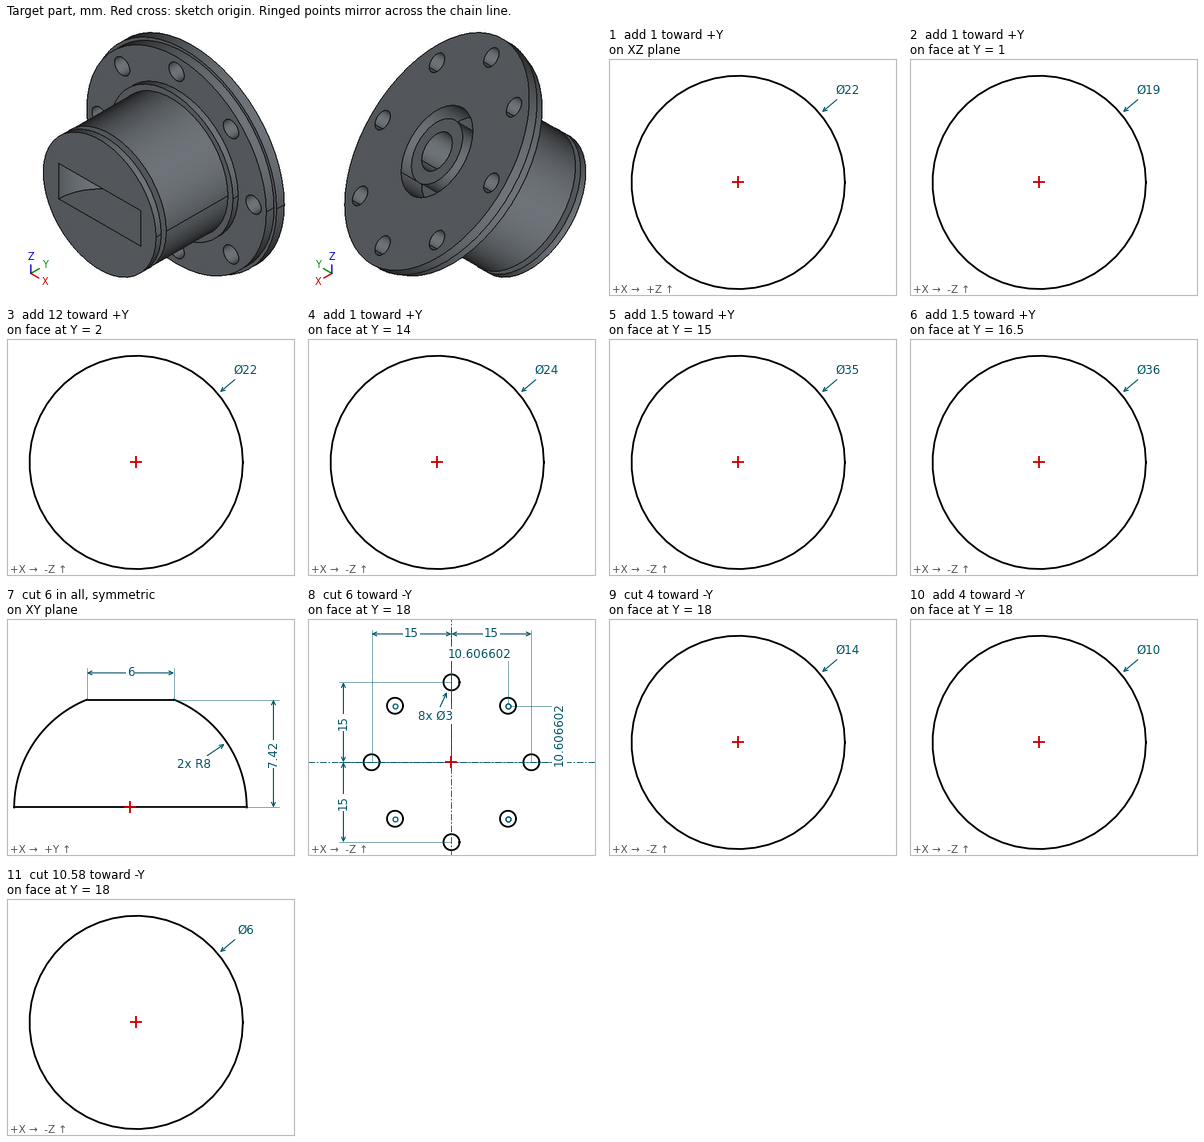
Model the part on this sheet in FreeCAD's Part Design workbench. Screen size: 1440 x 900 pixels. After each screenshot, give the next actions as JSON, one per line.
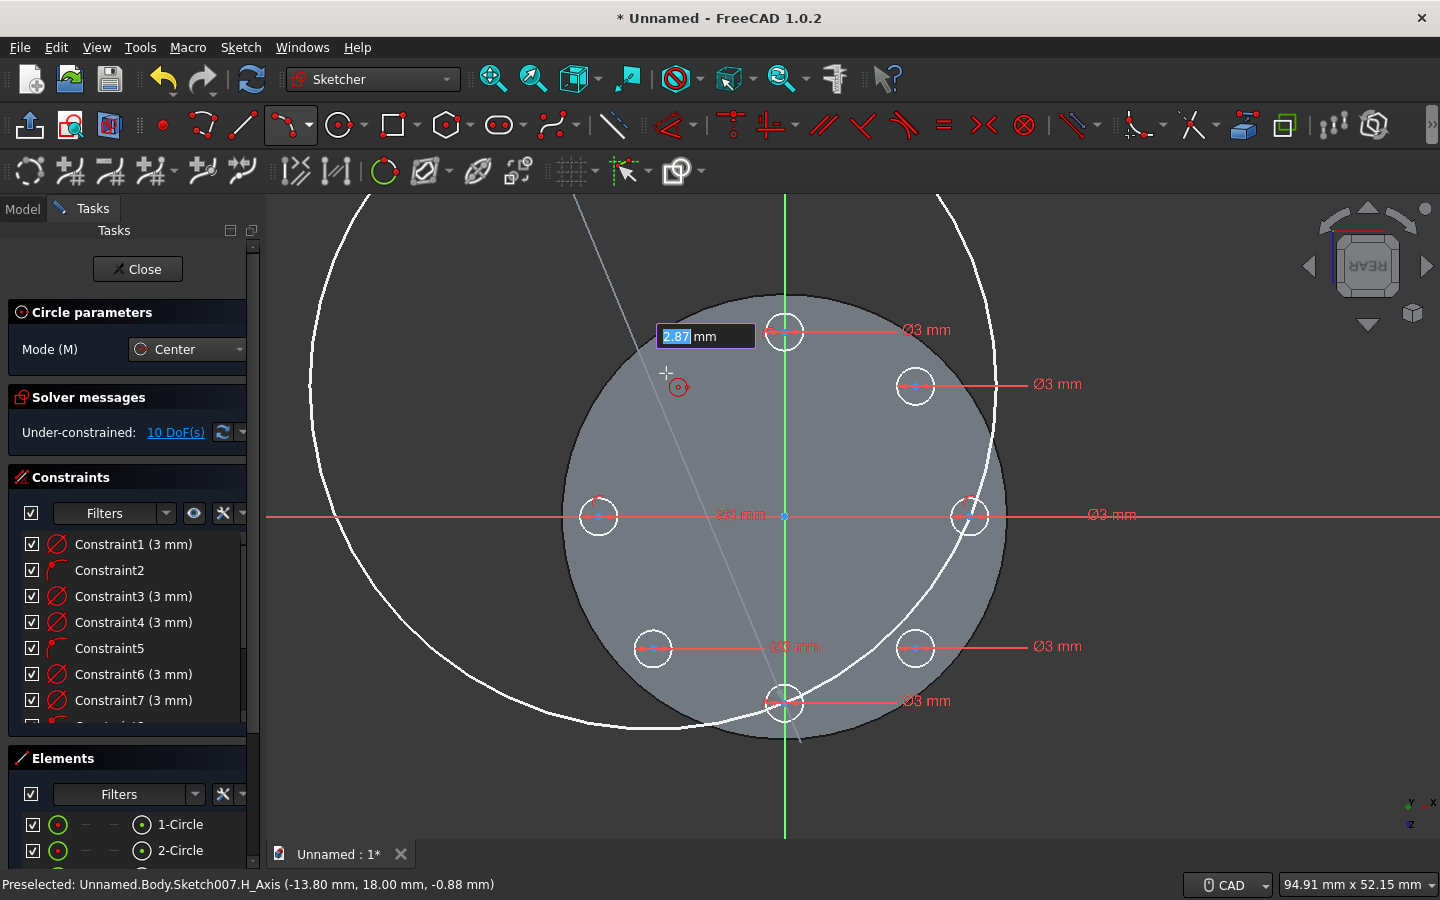
{"action": "type", "text": "3"}
{"action": "key", "text": "Return"}
{"action": "key", "text": "Escape"}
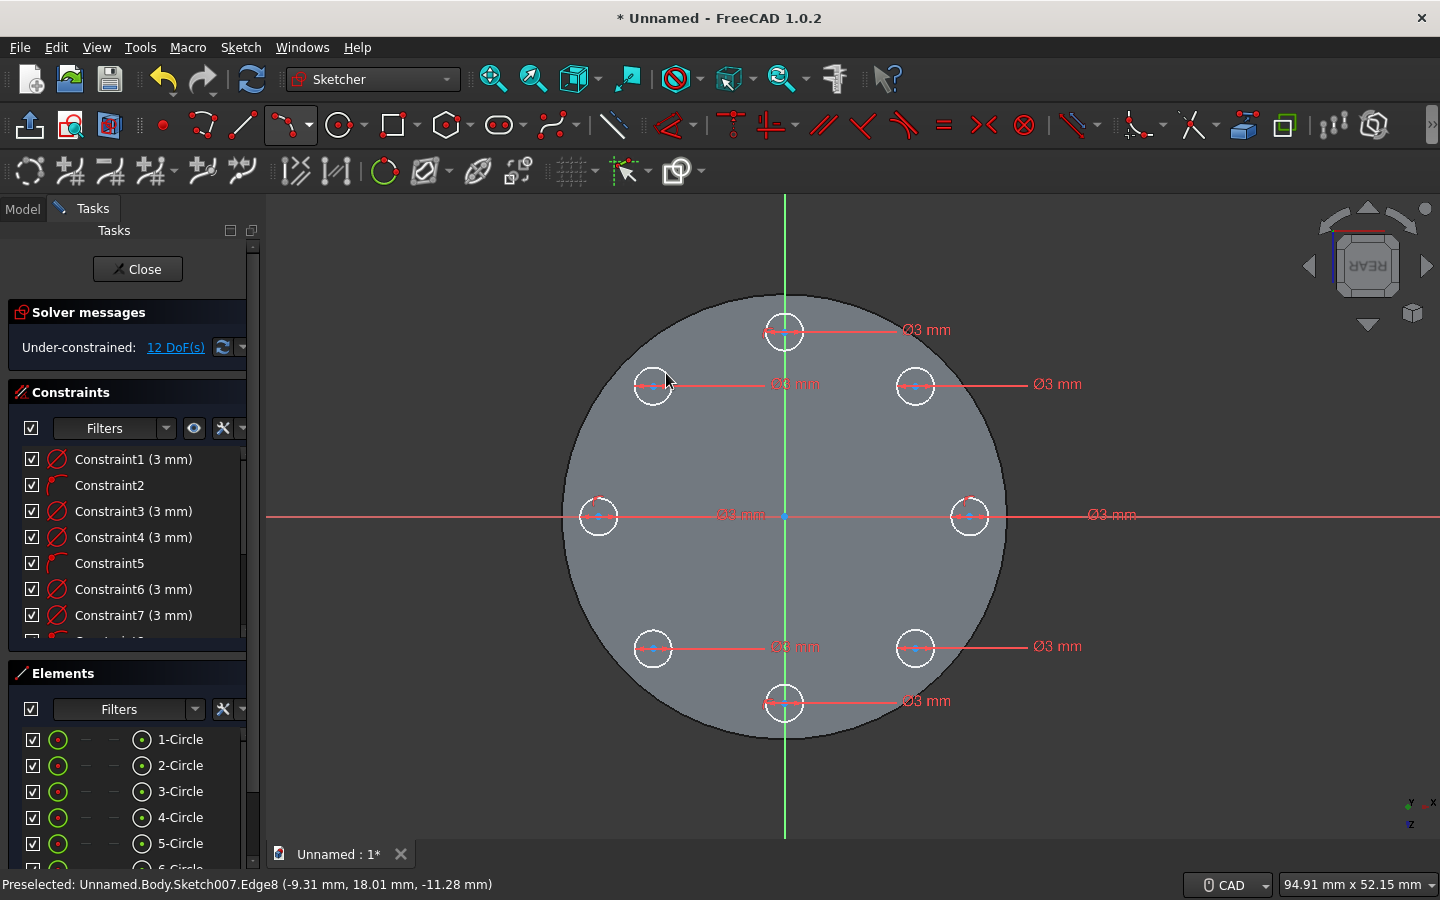
{"action": "left_click", "coordinate": [916, 386]}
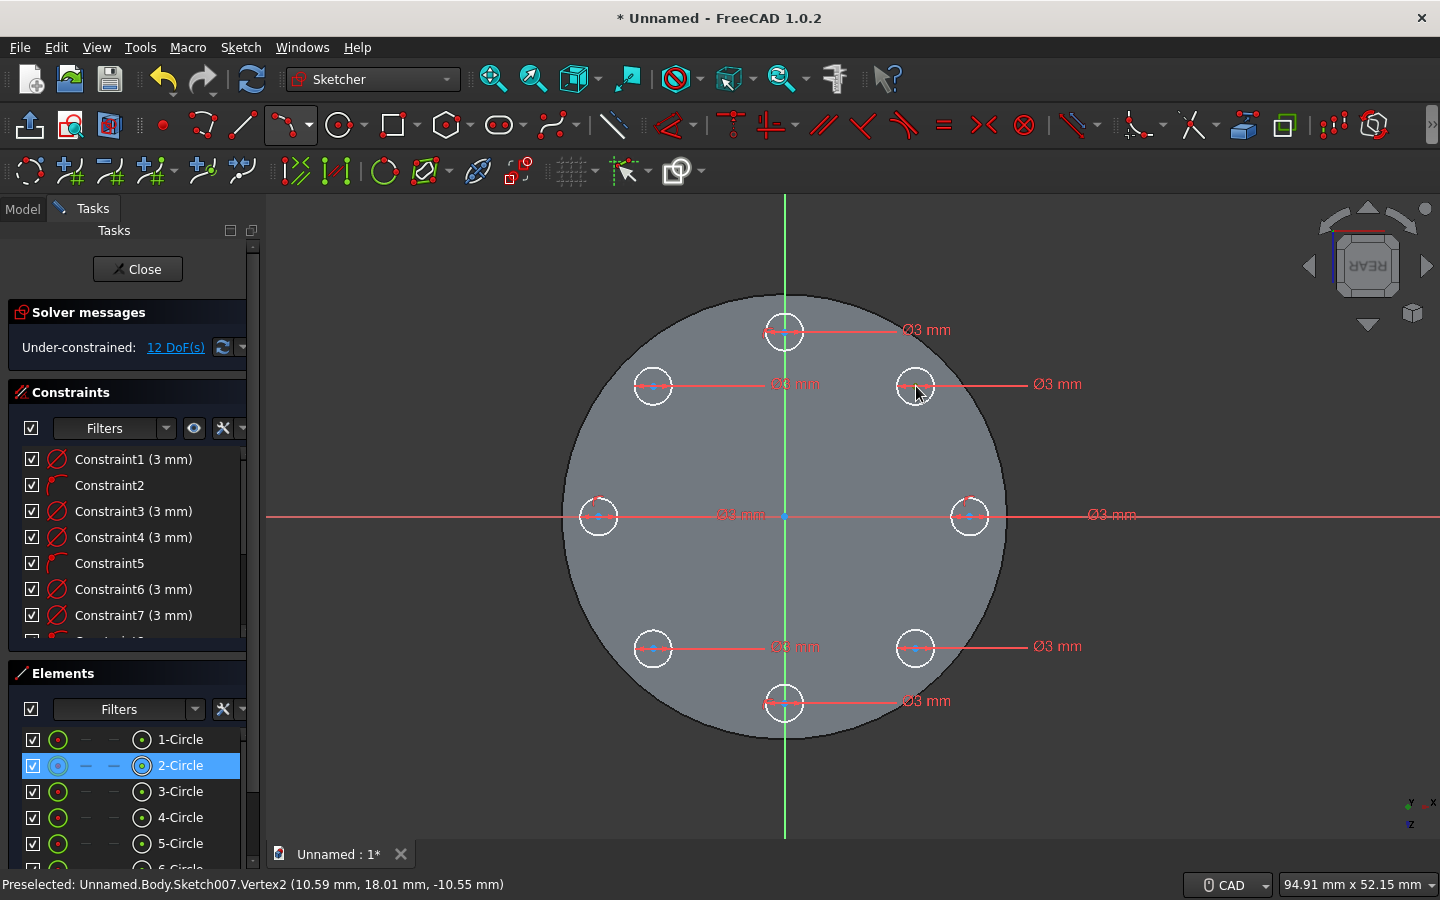
{"action": "left_click", "coordinate": [916, 648]}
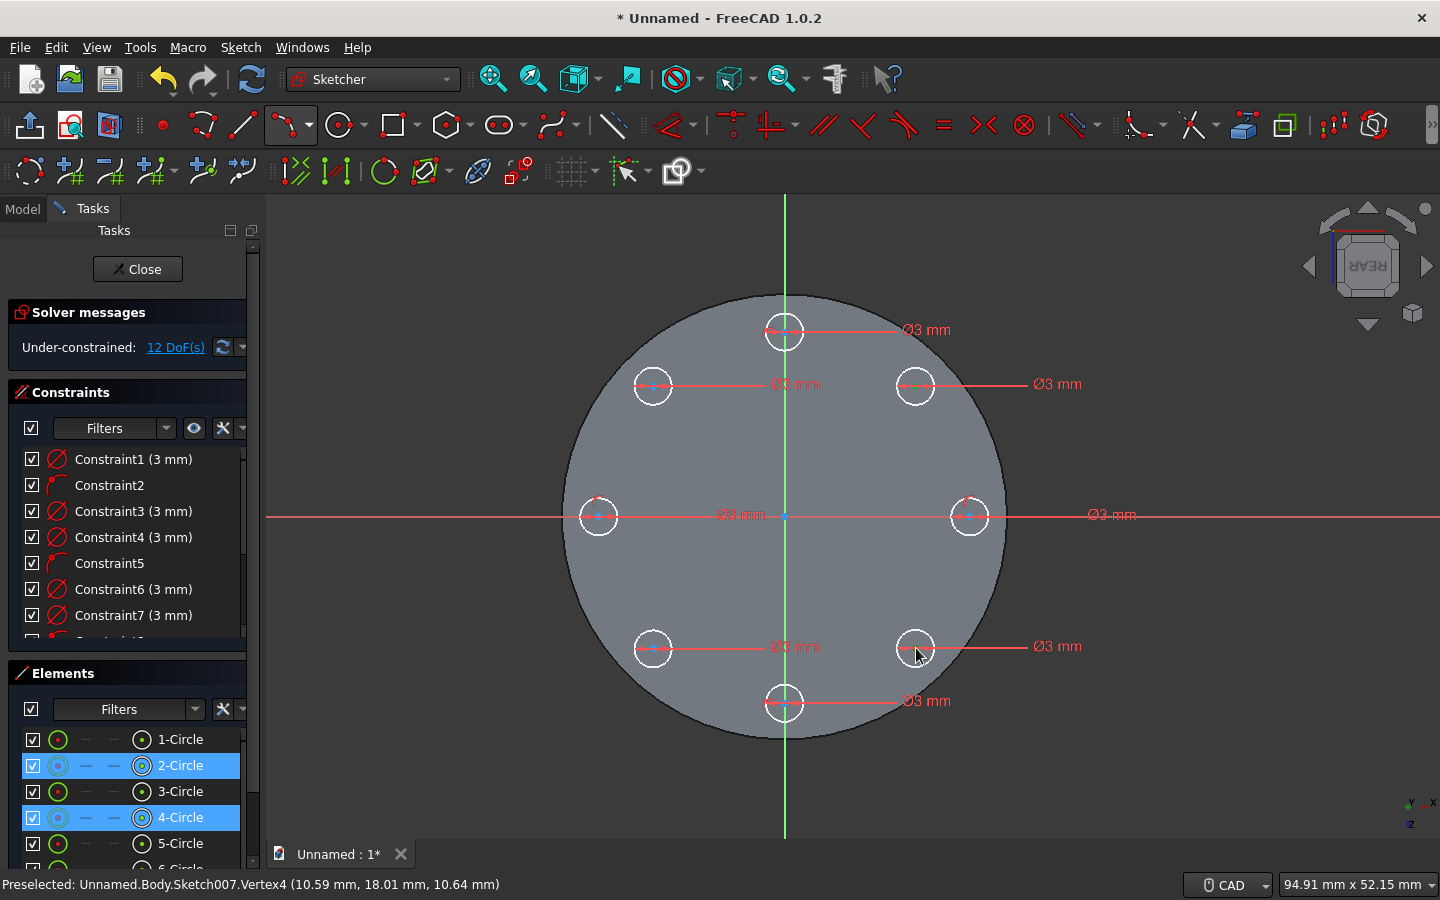
{"action": "left_click", "coordinate": [364, 517]}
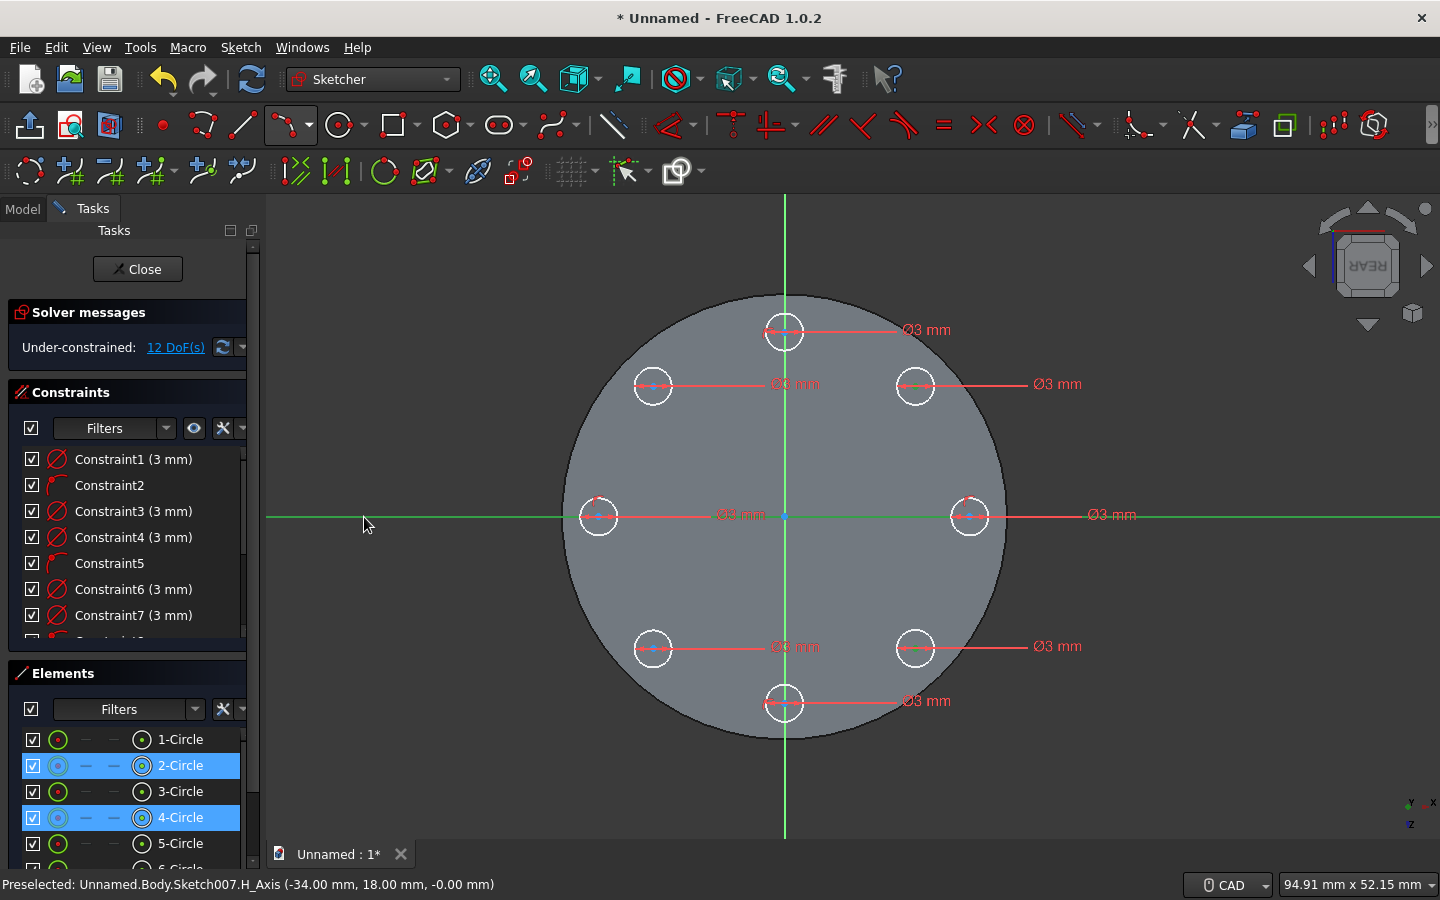
{"action": "left_click", "coordinate": [984, 126]}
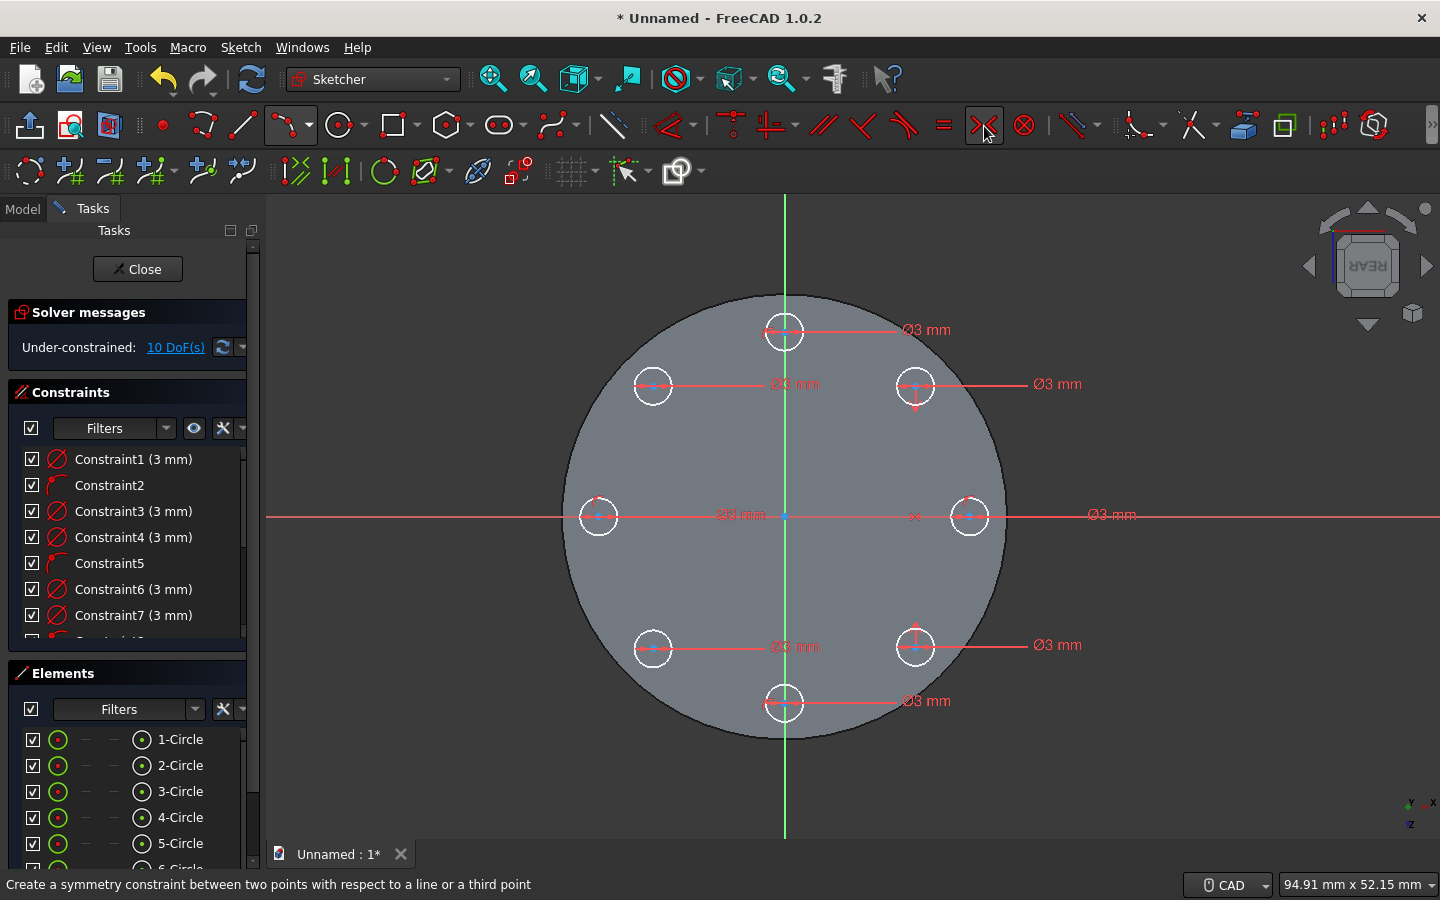
{"action": "left_click", "coordinate": [916, 647]}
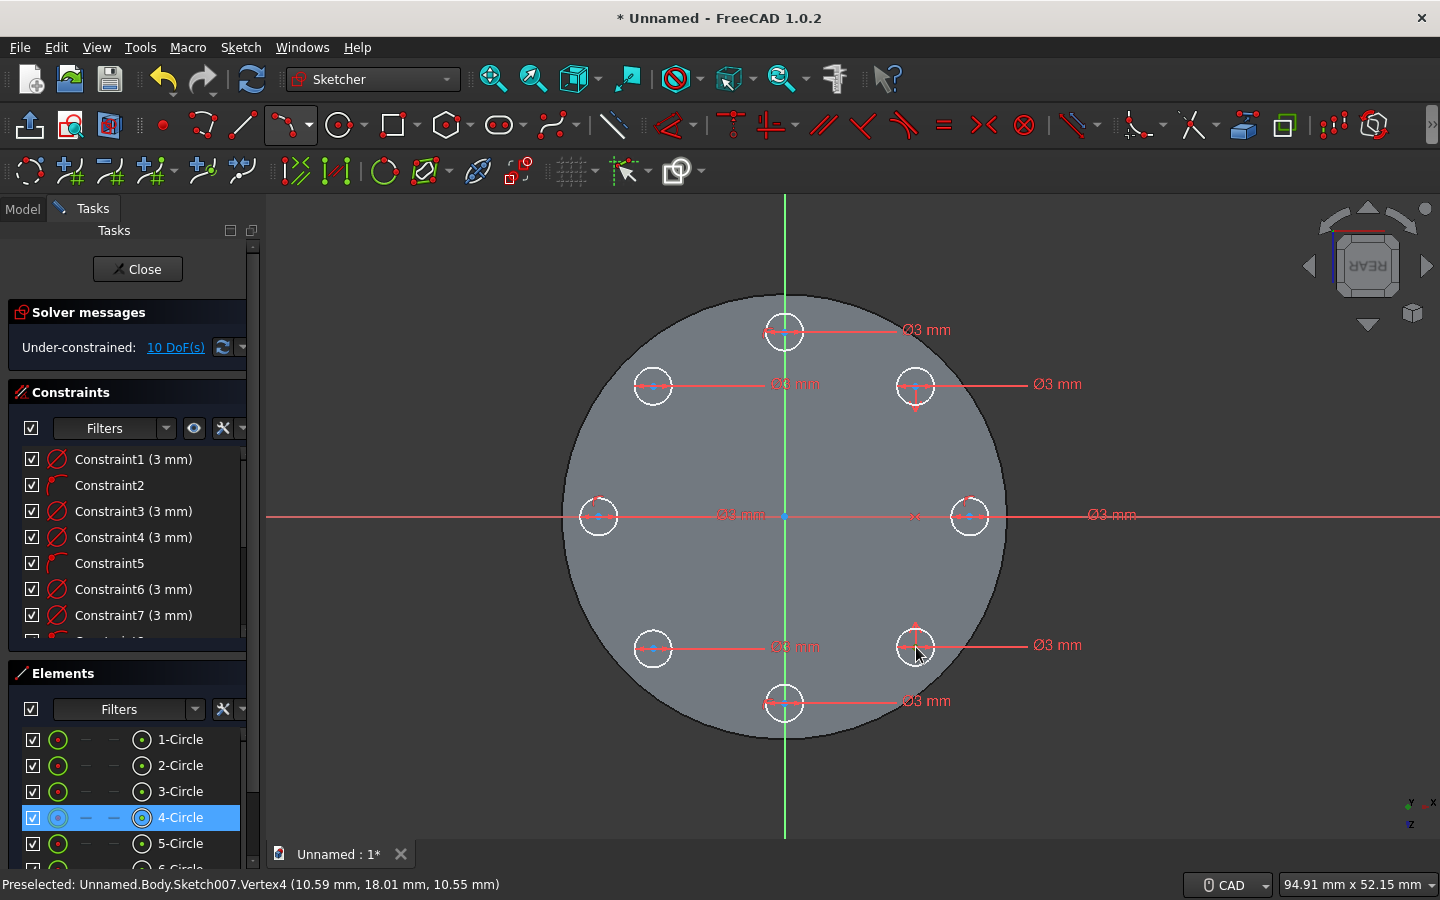
{"action": "left_click", "coordinate": [653, 649]}